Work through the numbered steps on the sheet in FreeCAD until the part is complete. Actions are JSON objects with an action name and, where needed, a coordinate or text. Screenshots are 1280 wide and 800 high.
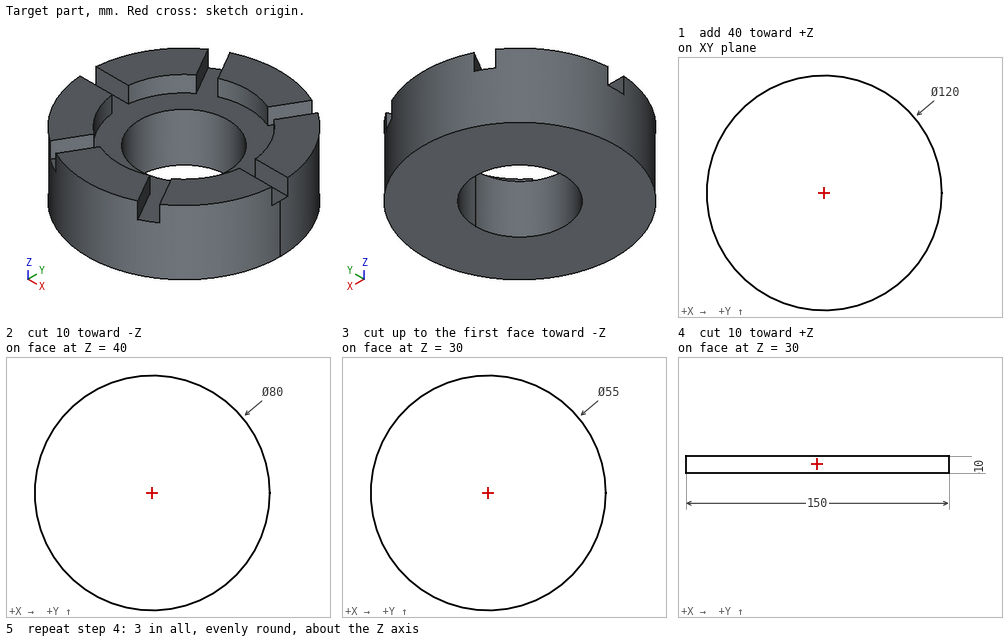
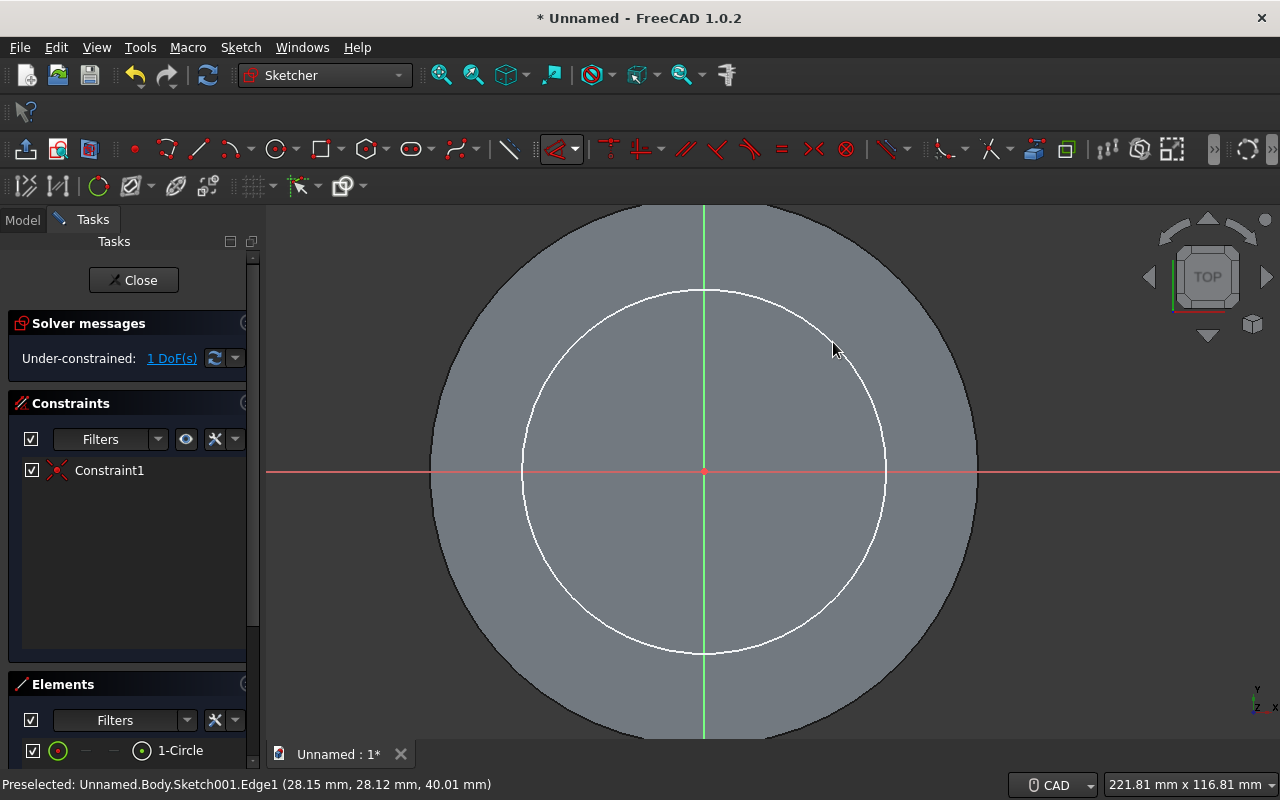
{"action": "key", "text": "d"}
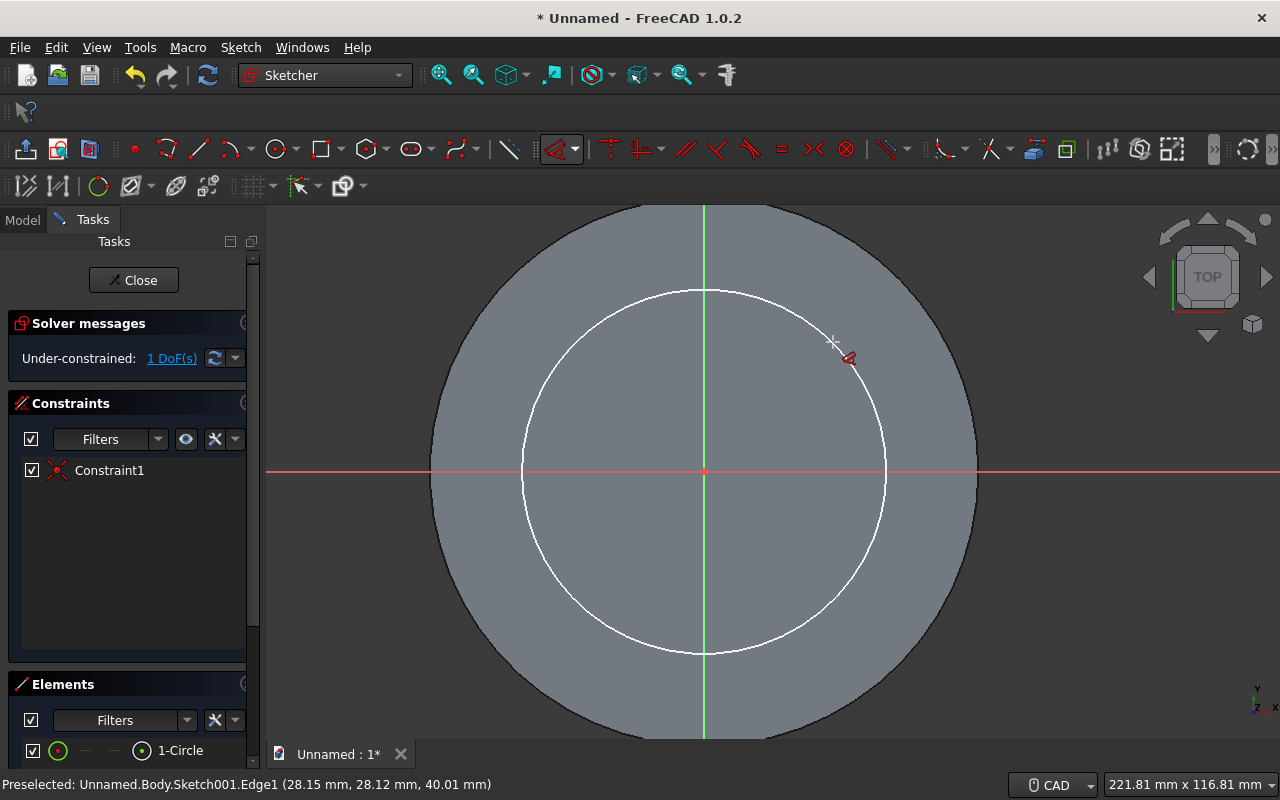
{"action": "left_click", "coordinate": [833, 343]}
{"action": "left_click", "coordinate": [856, 320]}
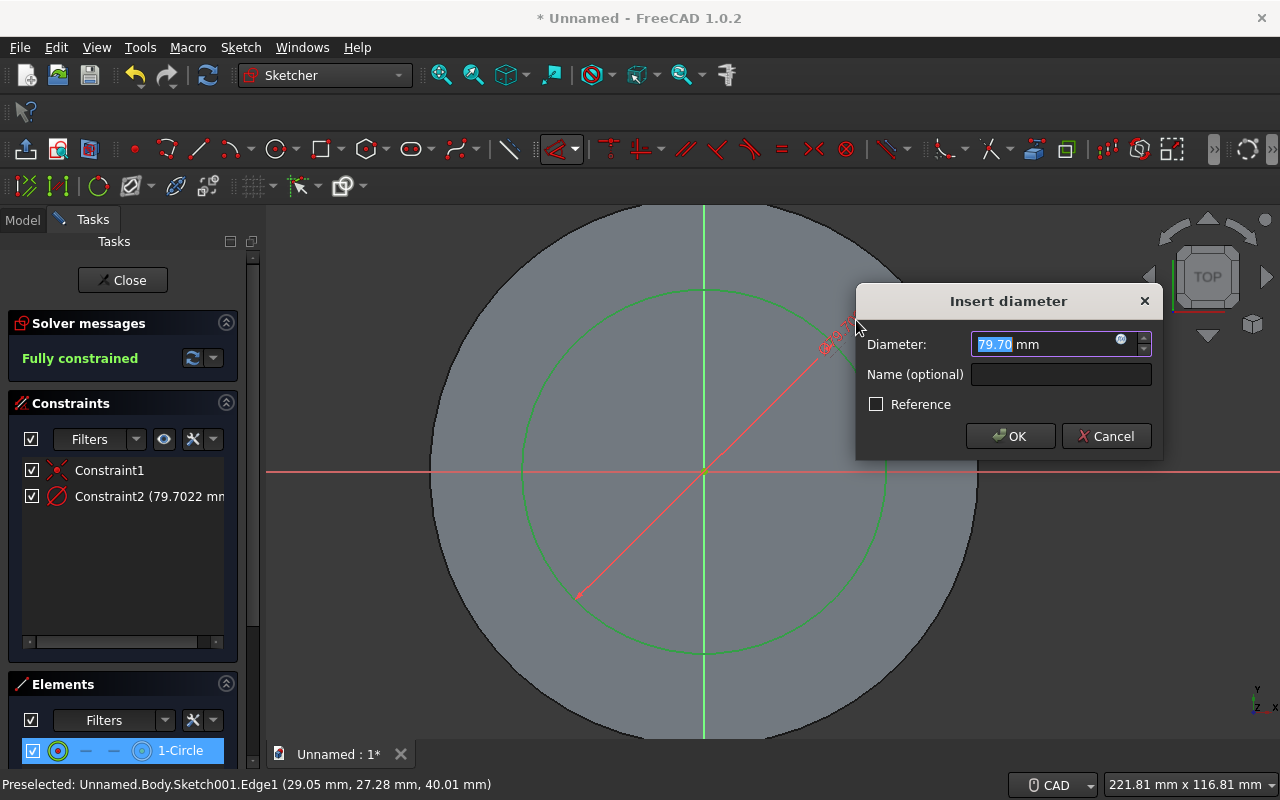
{"action": "type", "text": "80"}
{"action": "key", "text": "Return"}
{"action": "key", "text": "Escape"}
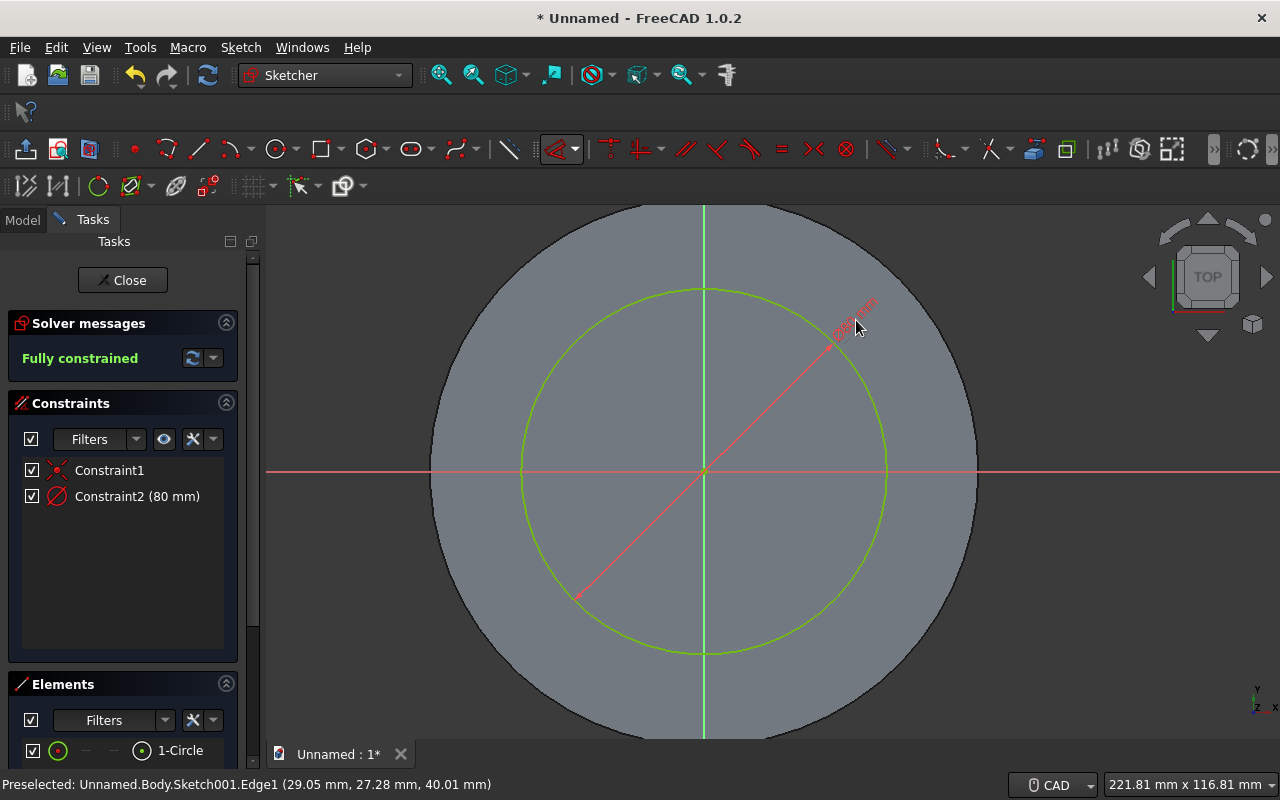
{"action": "left_click", "coordinate": [123, 280]}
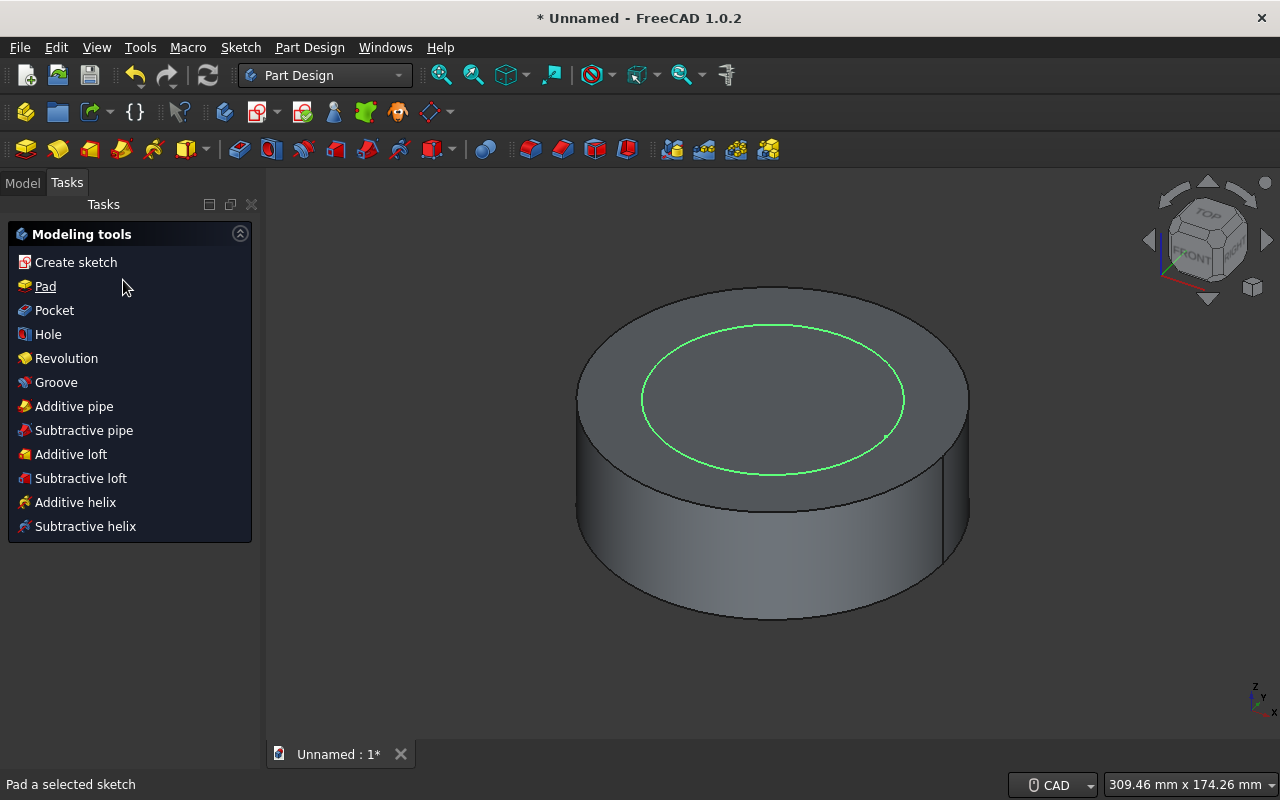
{"action": "left_click", "coordinate": [240, 150]}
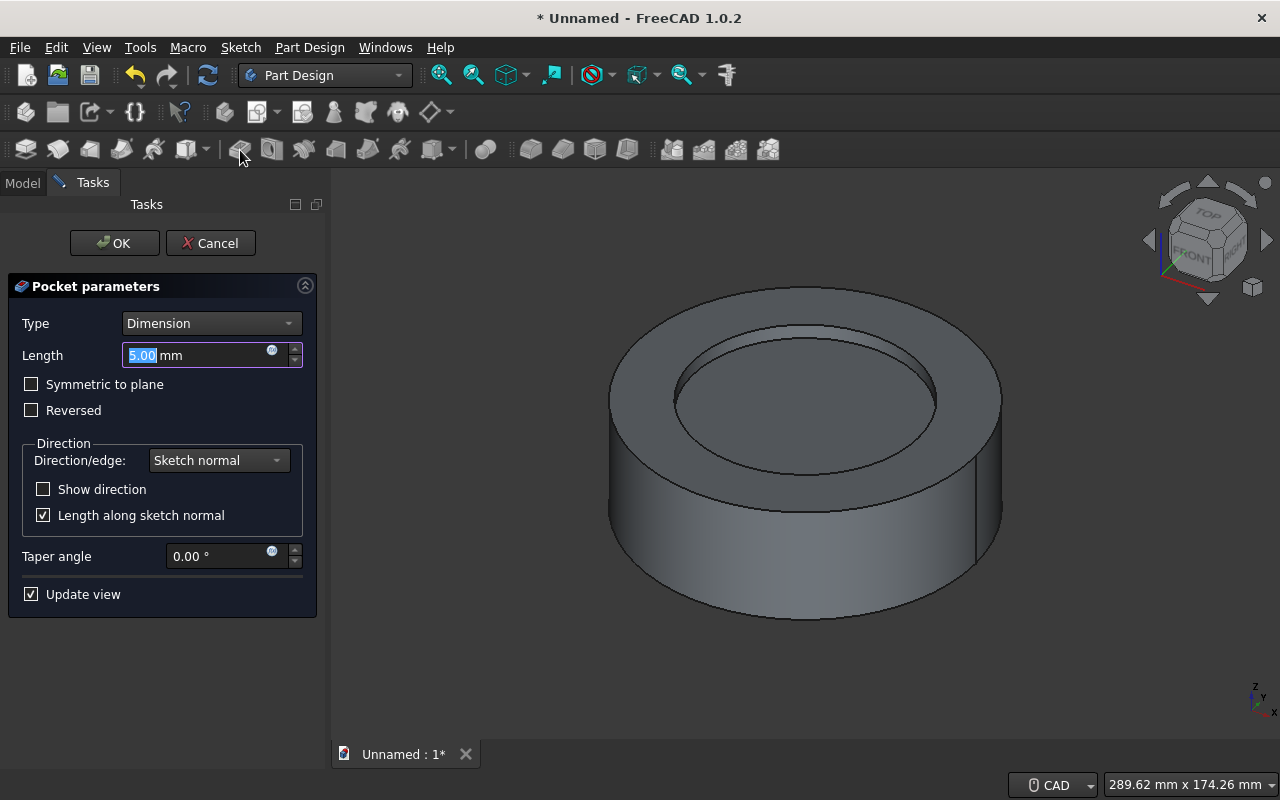
{"action": "type", "text": "10"}
{"action": "key", "text": "Tab"}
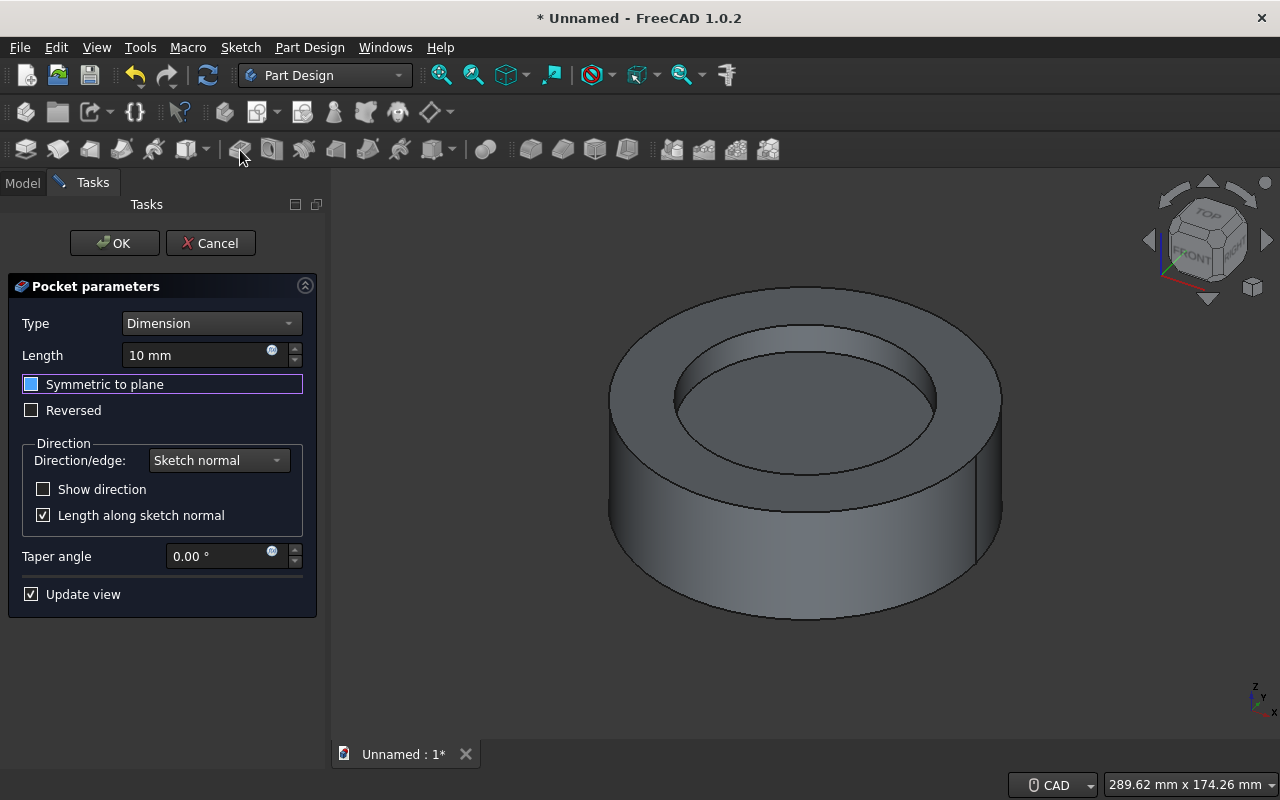
{"action": "left_click", "coordinate": [115, 243]}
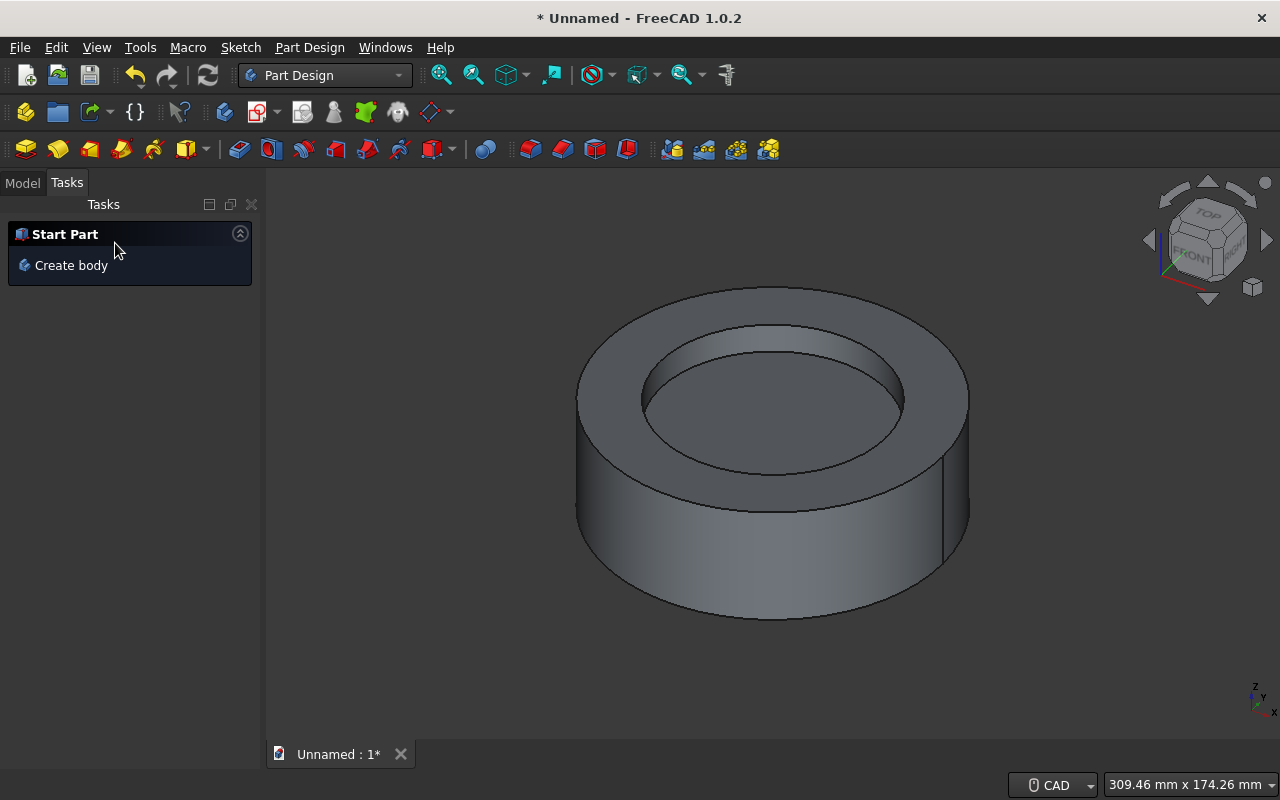
{"action": "left_click", "coordinate": [773, 426]}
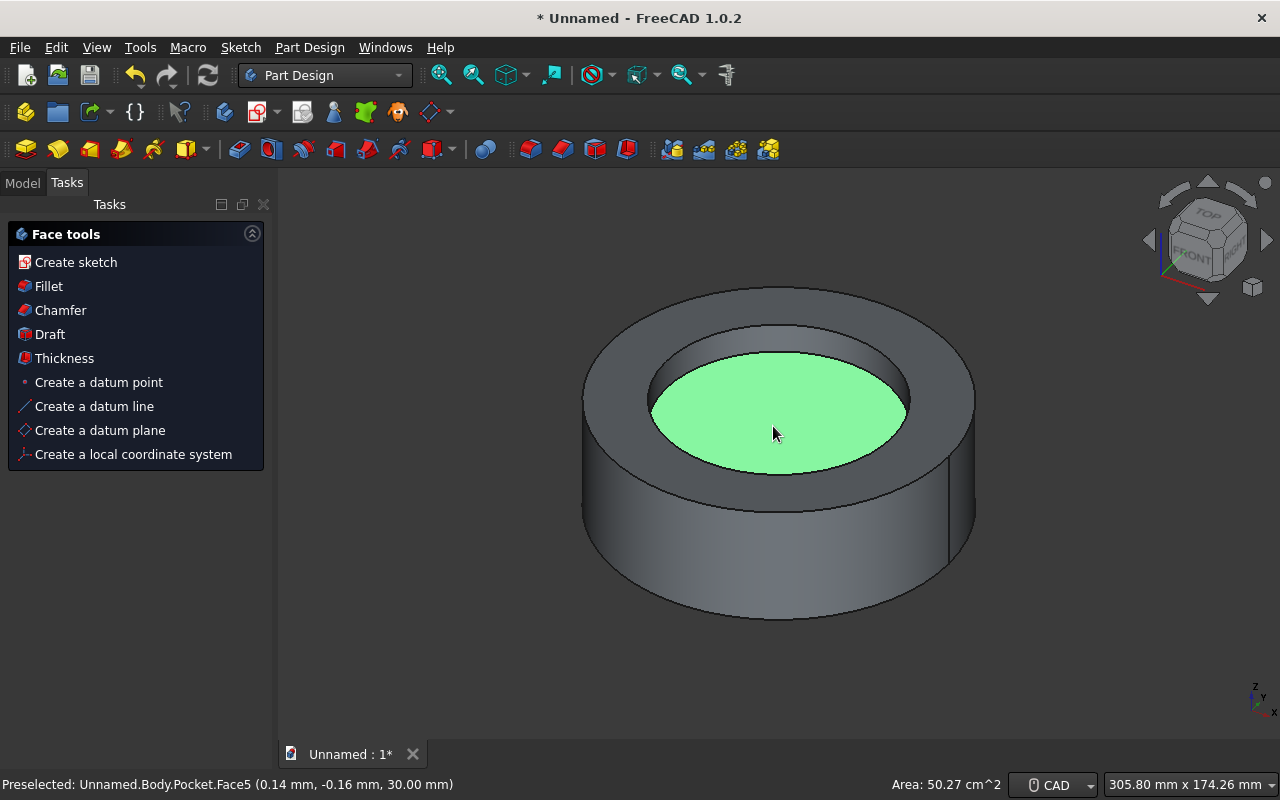
{"action": "left_click", "coordinate": [258, 112]}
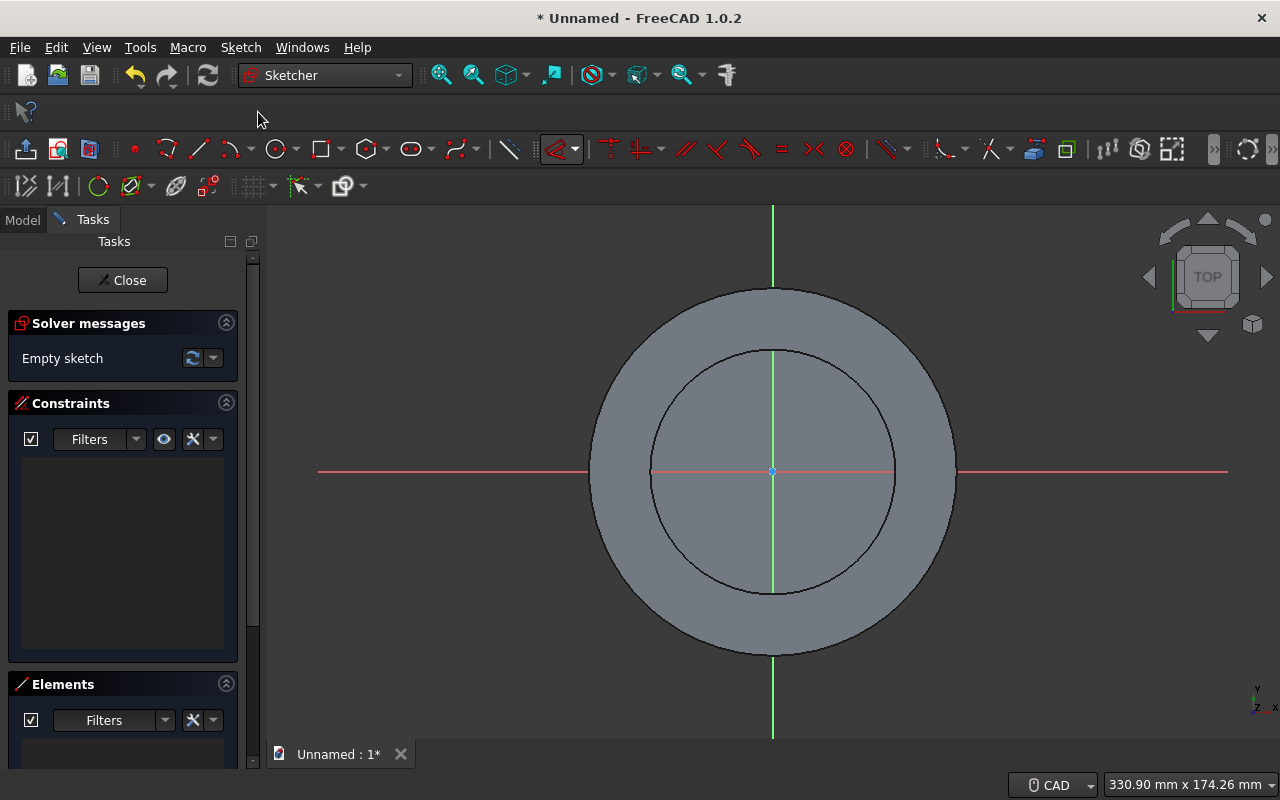
{"action": "scroll", "coordinate": [856, 472], "scroll_direction": "up", "scroll_amount": 3}